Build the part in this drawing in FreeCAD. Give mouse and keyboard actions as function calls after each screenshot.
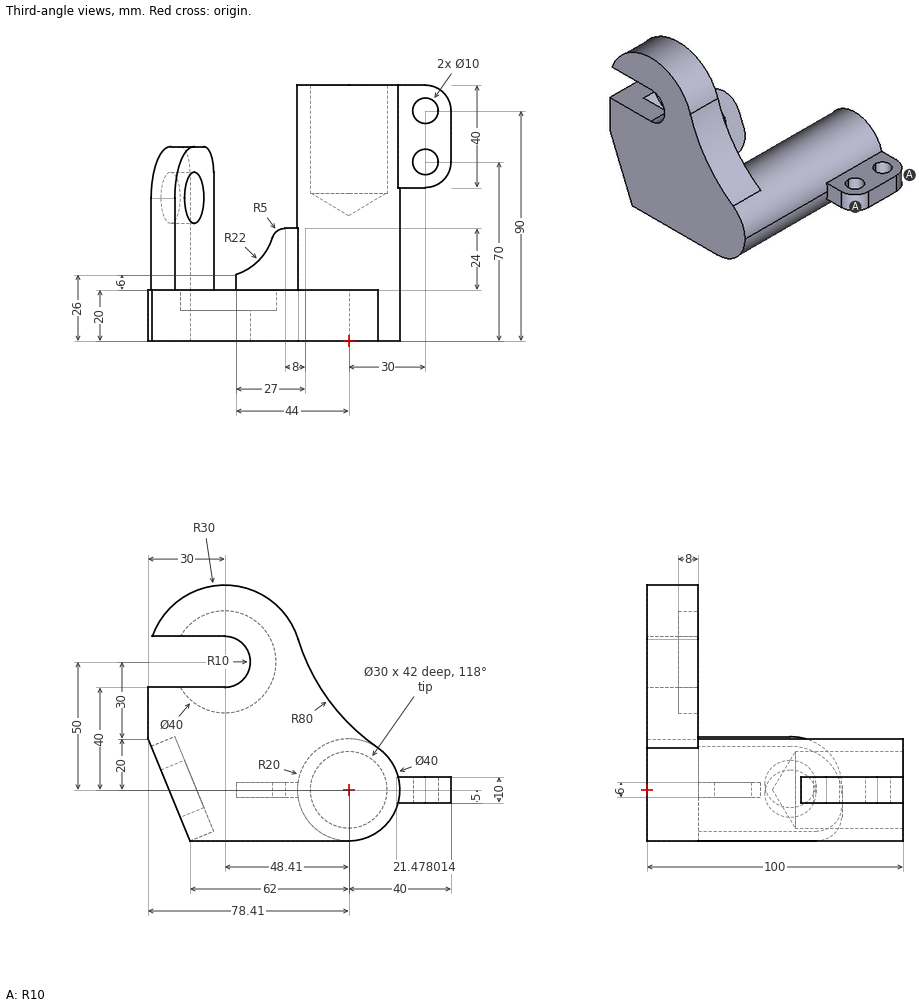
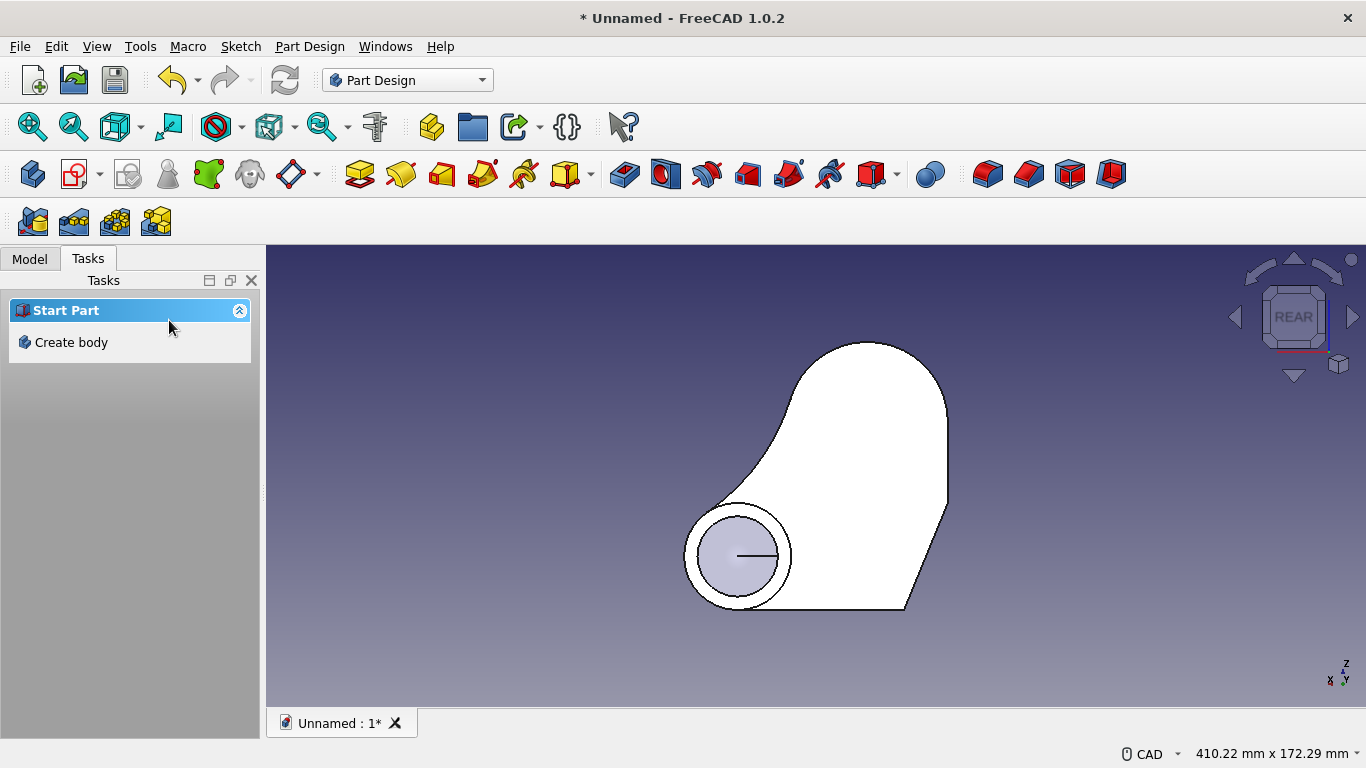
key(6)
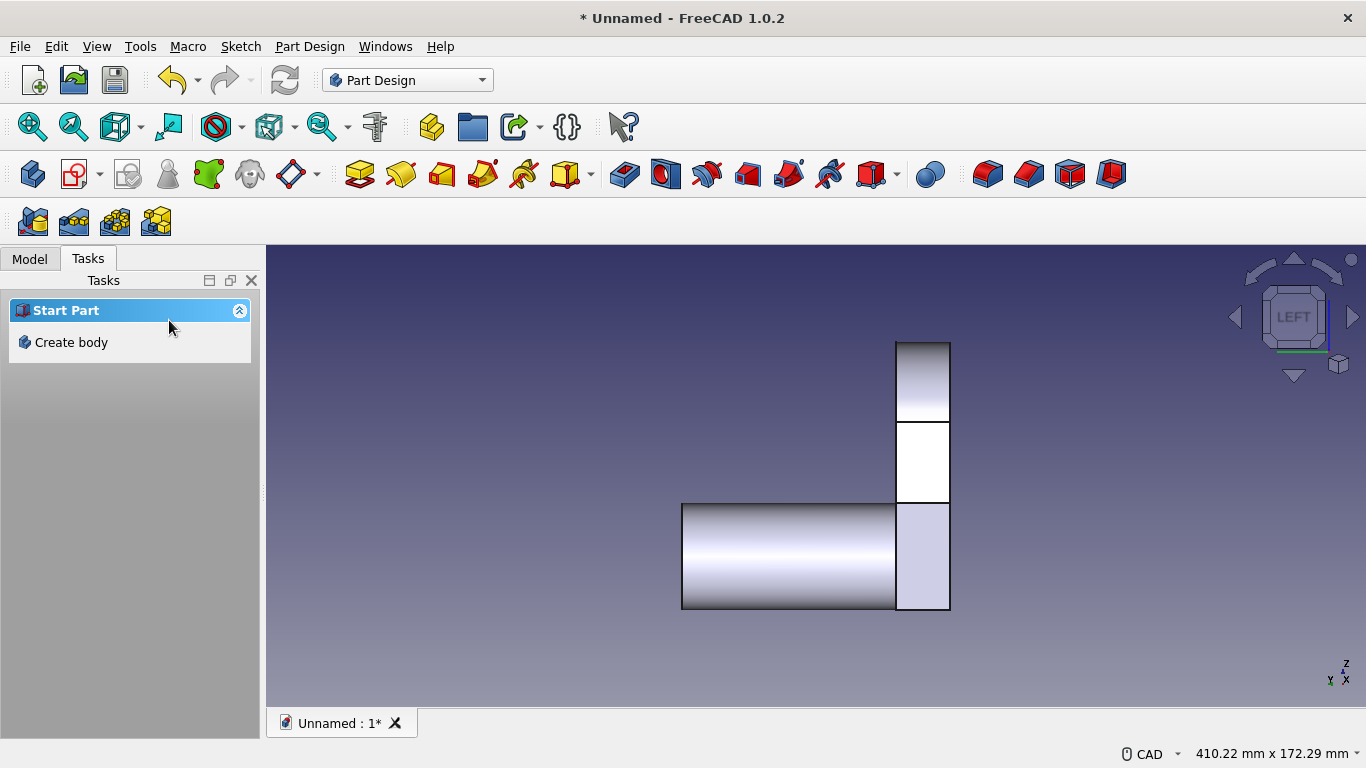
click(923, 571)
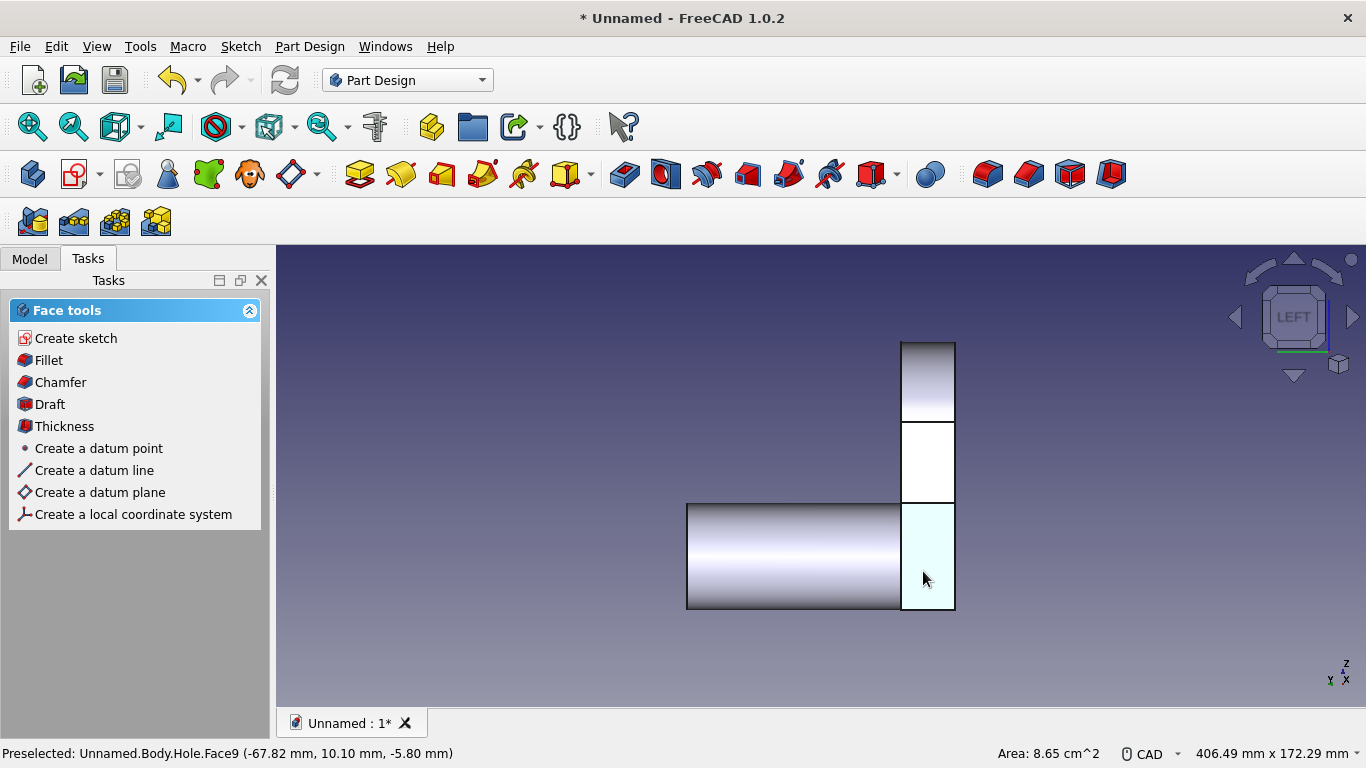
click(74, 174)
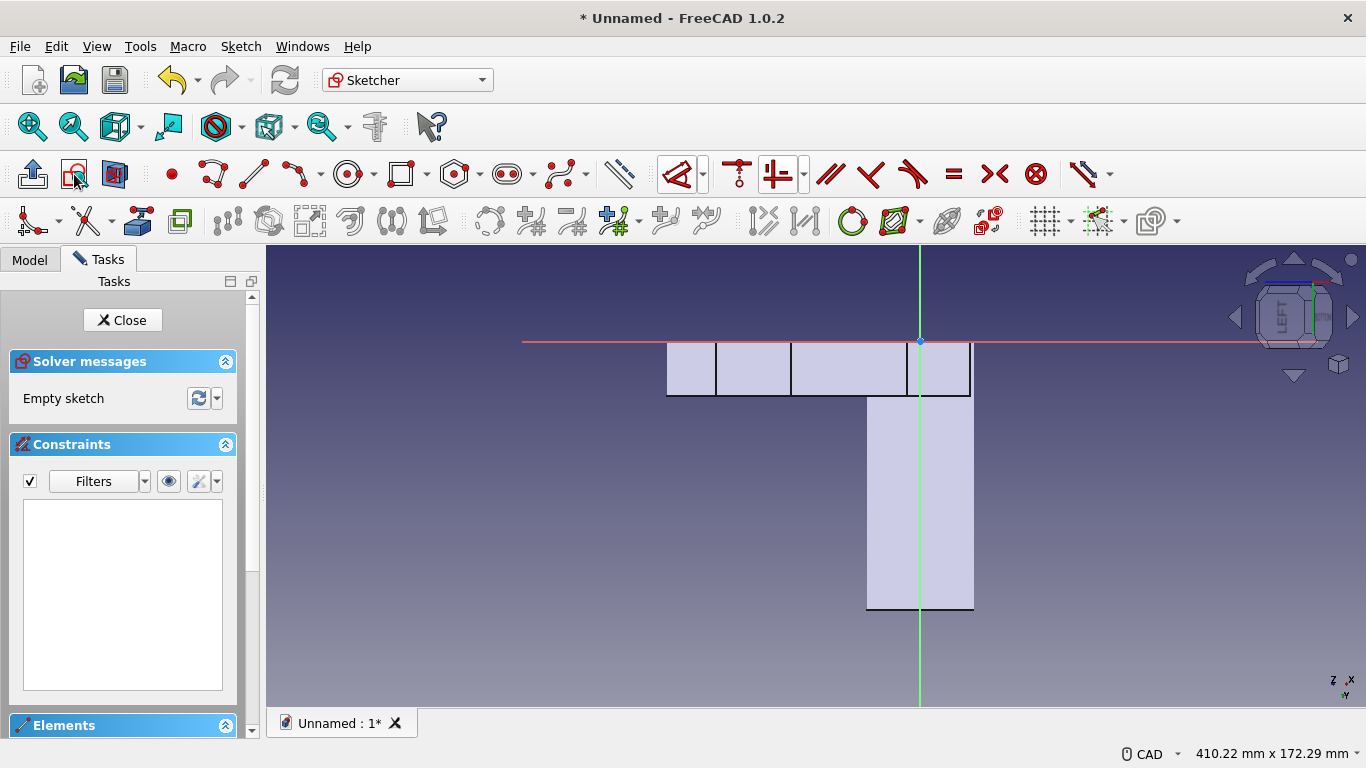
scroll(1088, 378, up, 2)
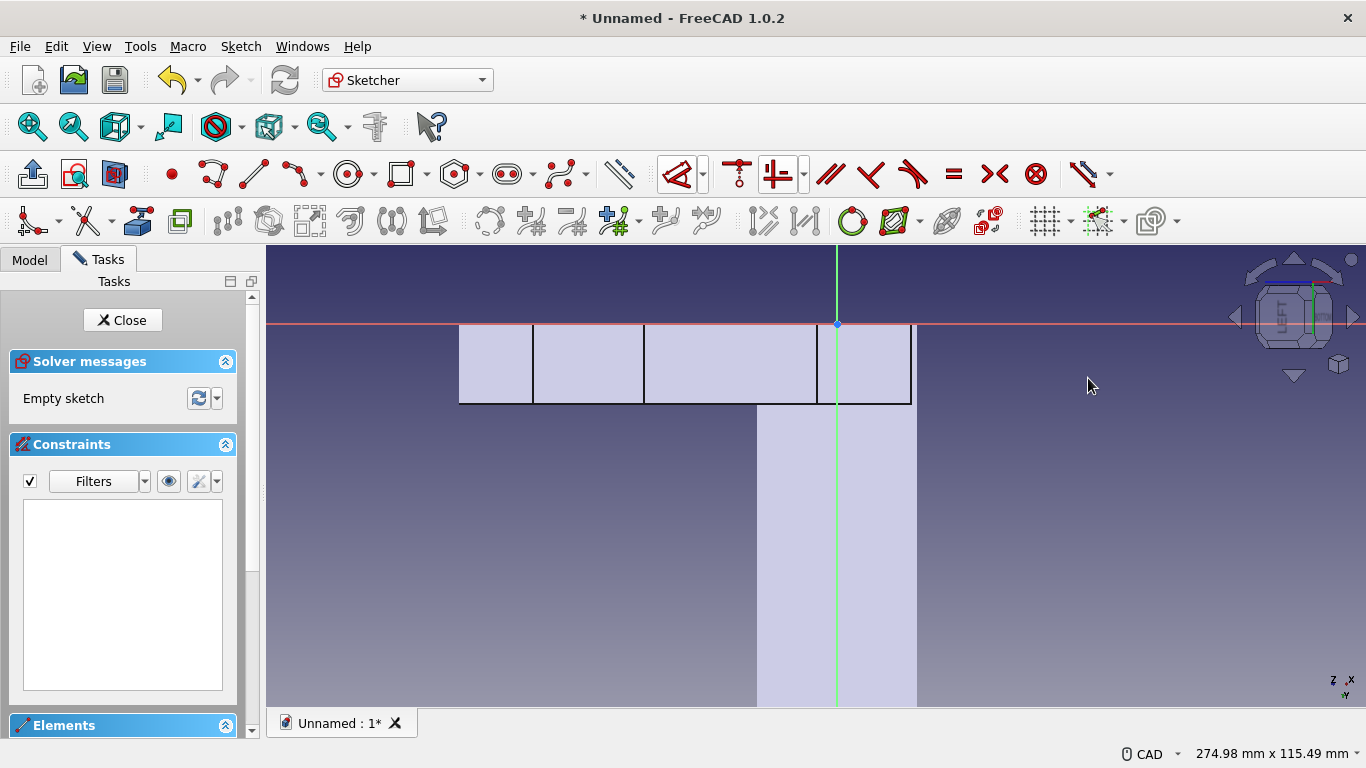
click(213, 174)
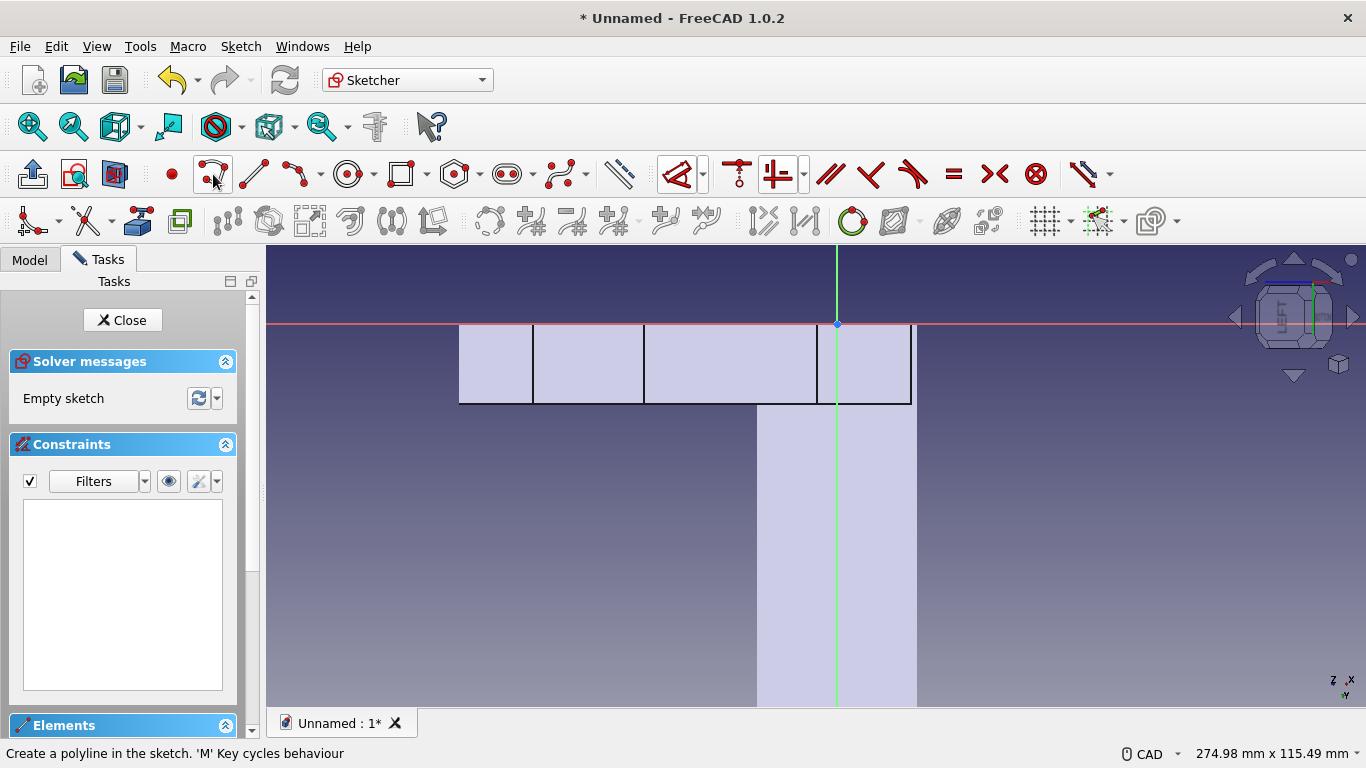
click(817, 588)
click(817, 404)
click(657, 404)
click(657, 548)
right_click(657, 548)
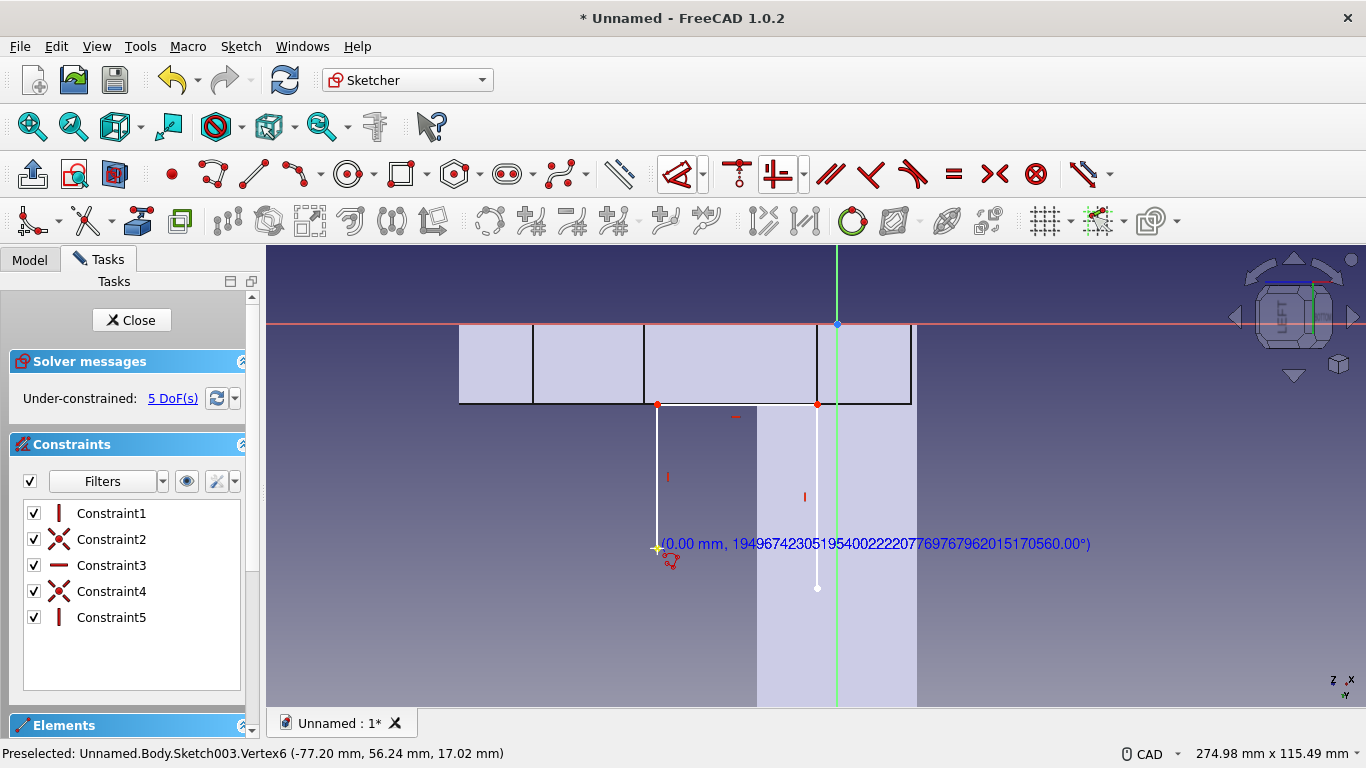
key(g)
key(l)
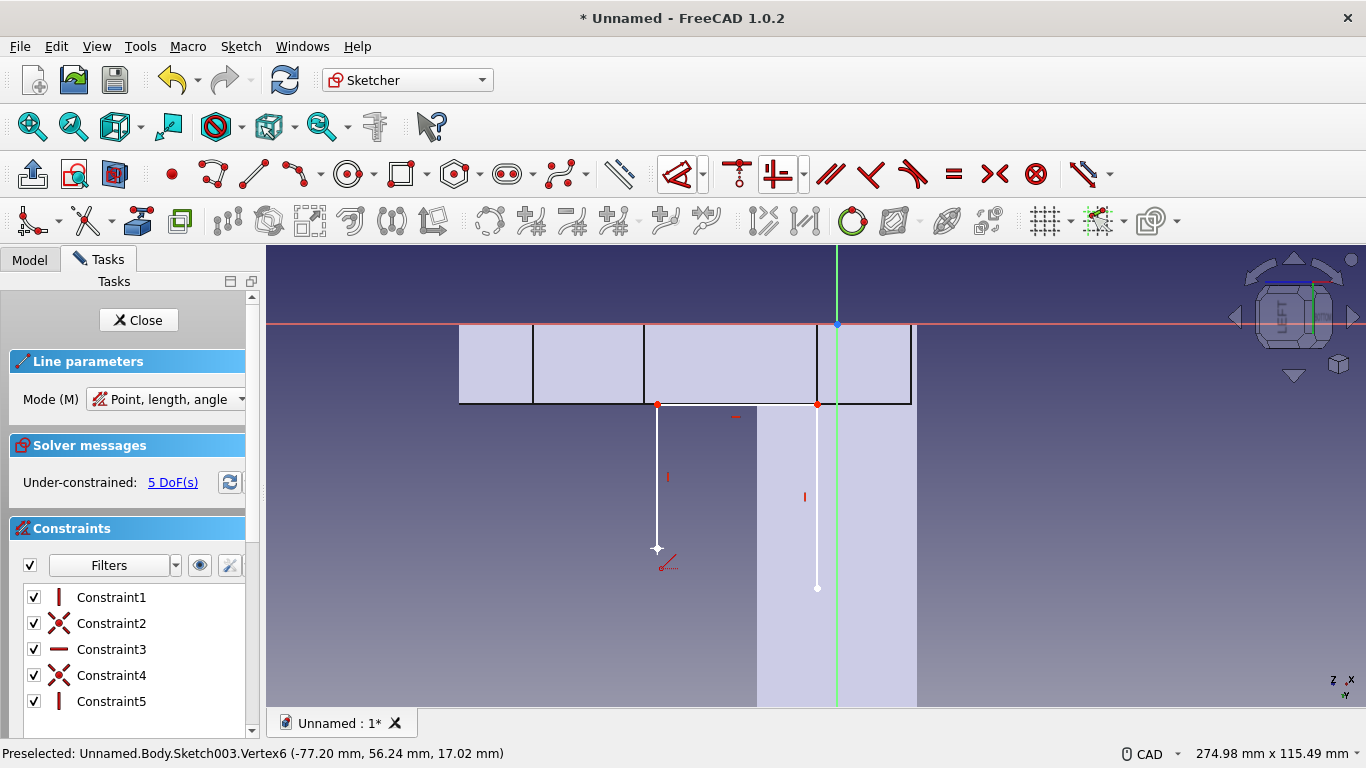
click(737, 628)
click(777, 628)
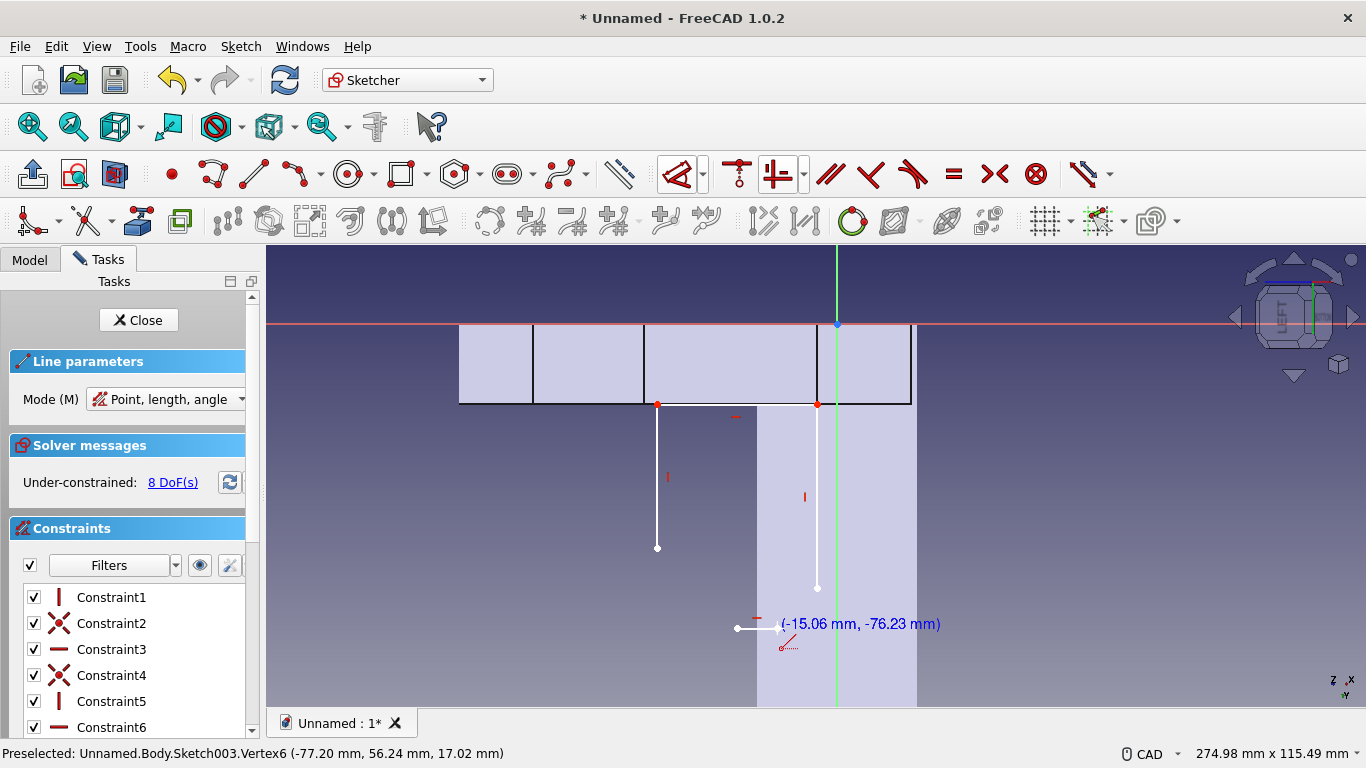
key(g)
key(3)
key(a)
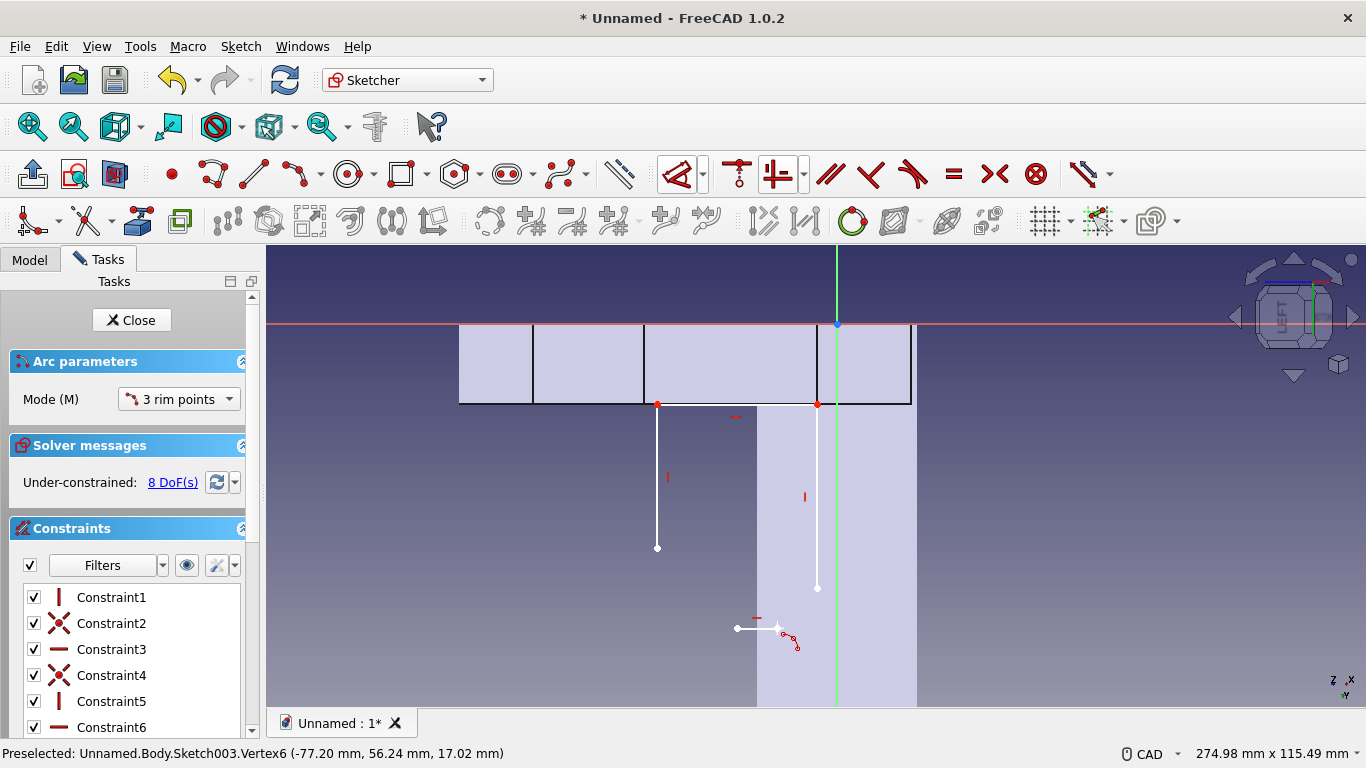
click(657, 549)
click(737, 629)
click(681, 605)